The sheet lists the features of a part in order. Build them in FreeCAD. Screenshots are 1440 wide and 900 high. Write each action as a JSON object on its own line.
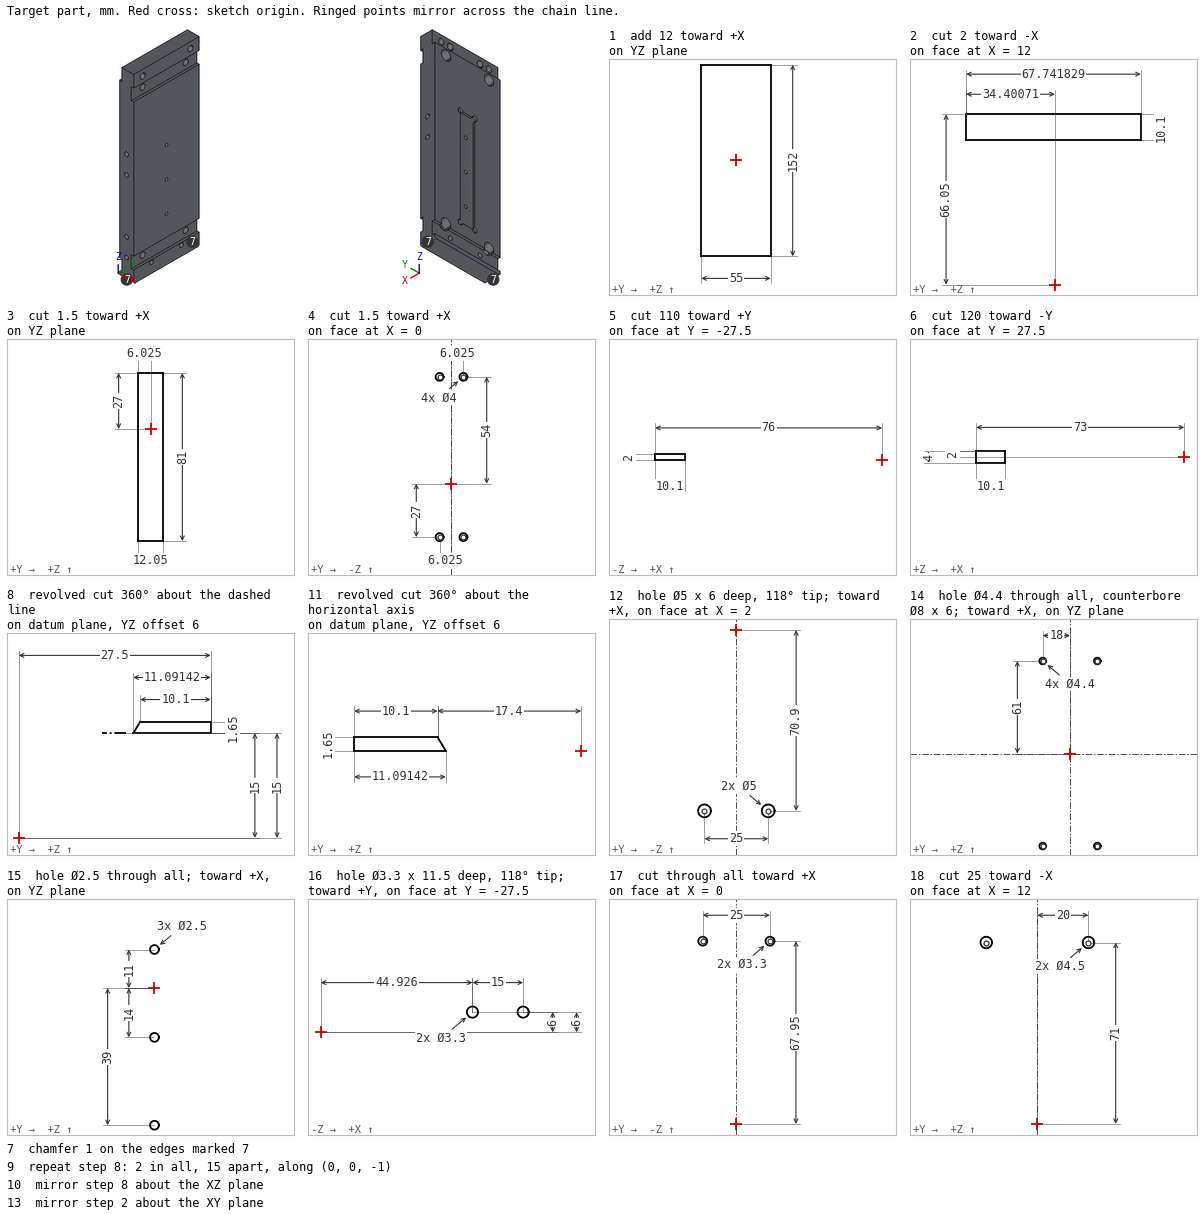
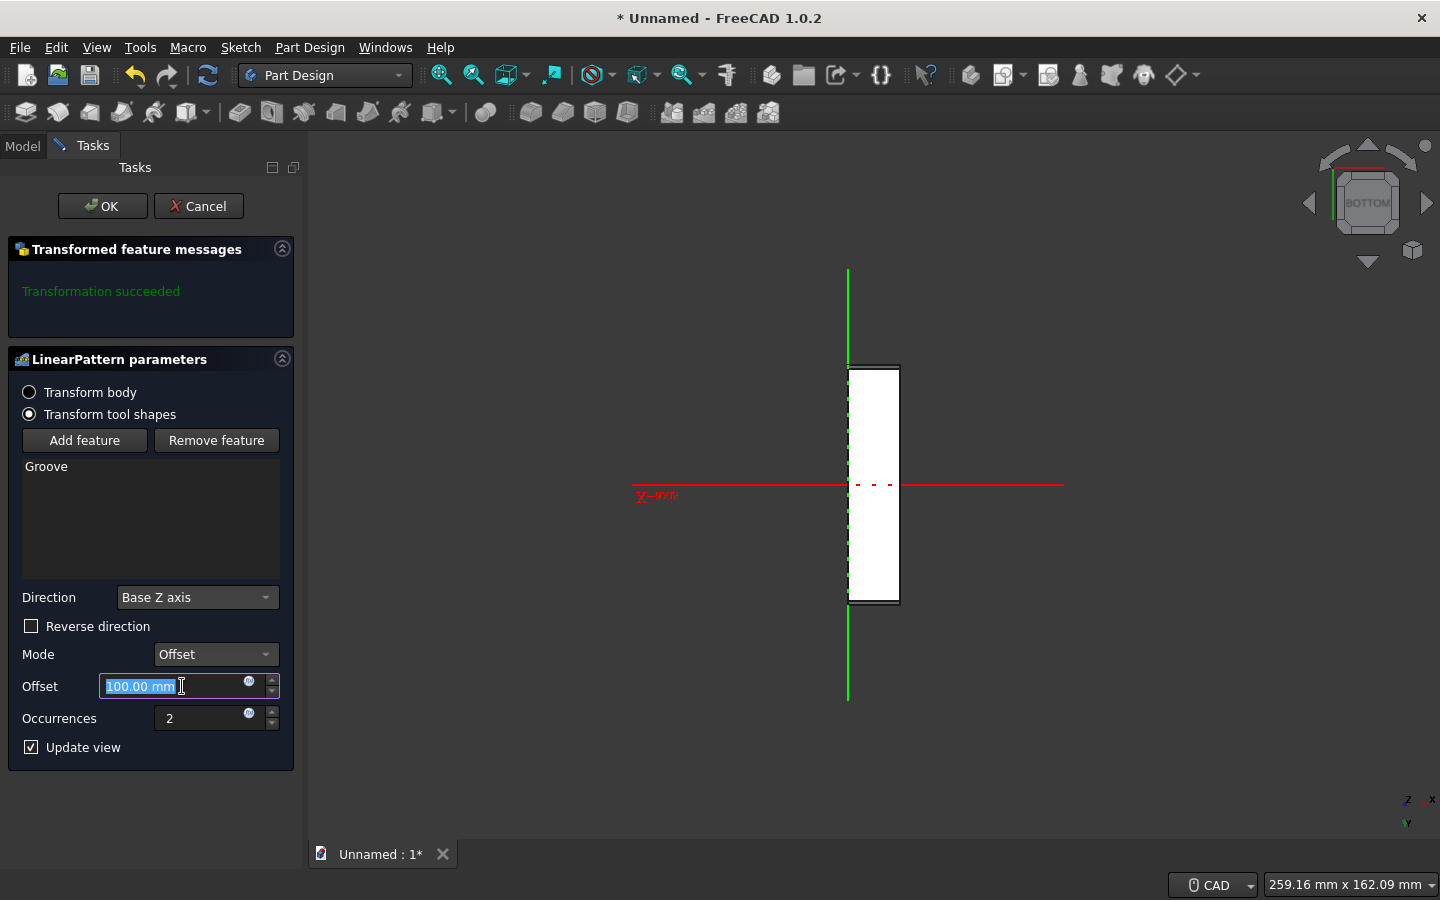
{"action": "type", "text": "15"}
{"action": "key", "text": "Tab"}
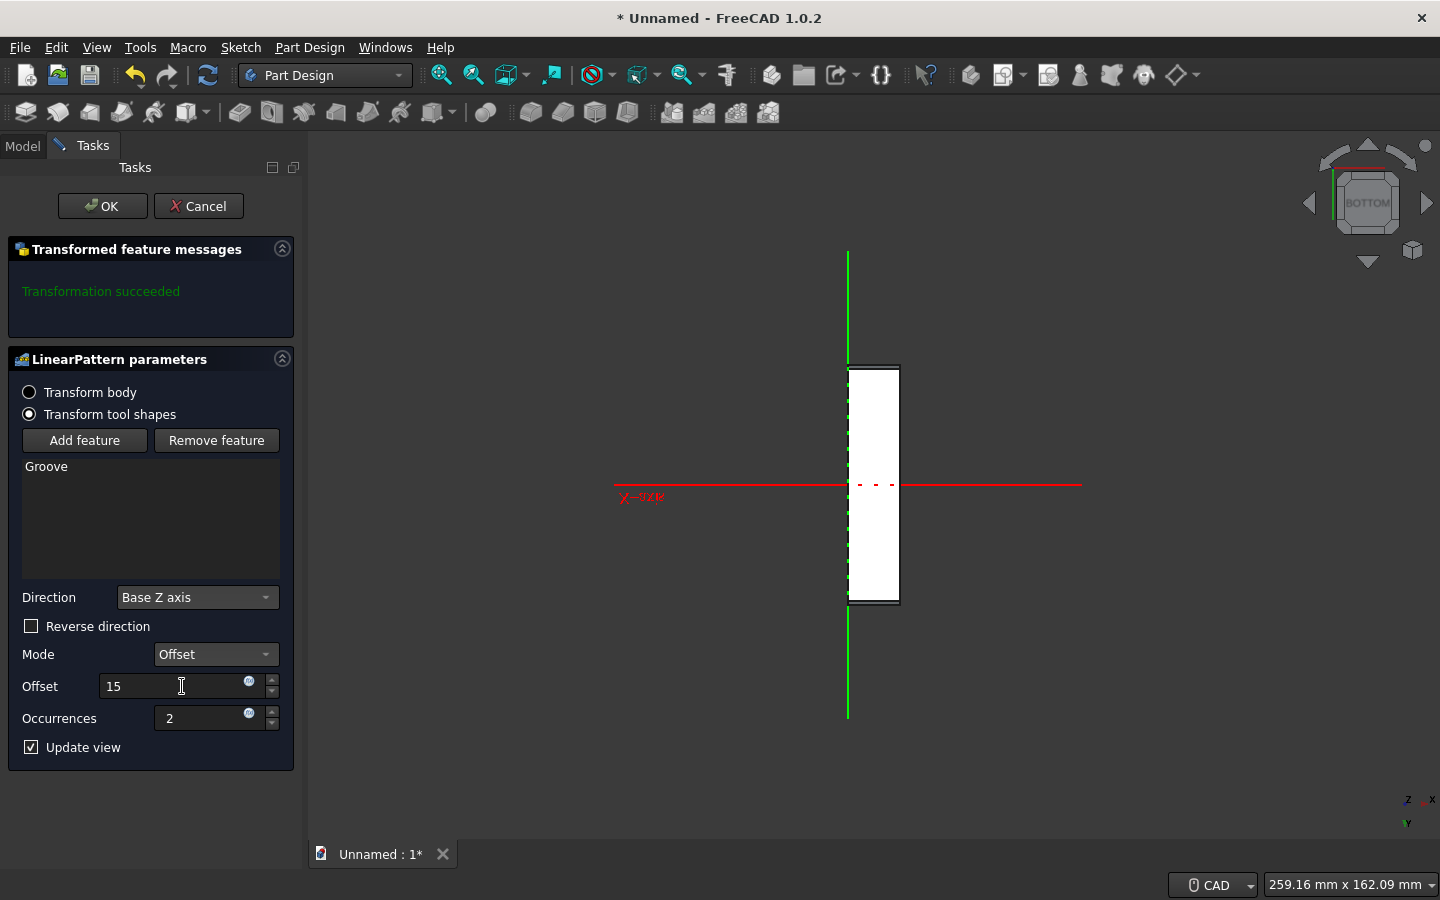
{"action": "triple_click", "coordinate": [209, 718]}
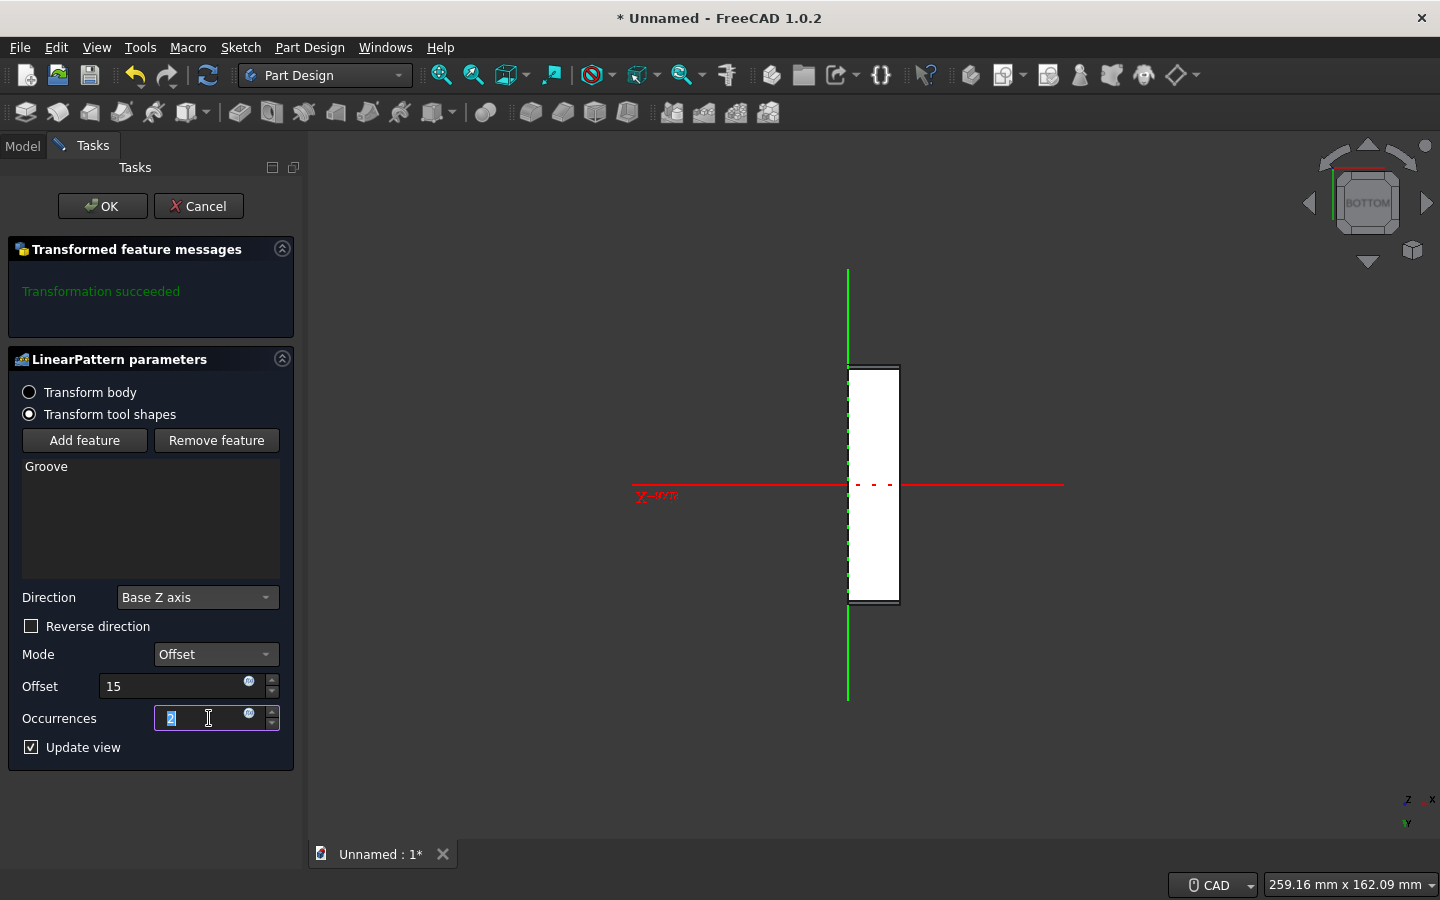
{"action": "type", "text": "2"}
{"action": "key", "text": "Tab"}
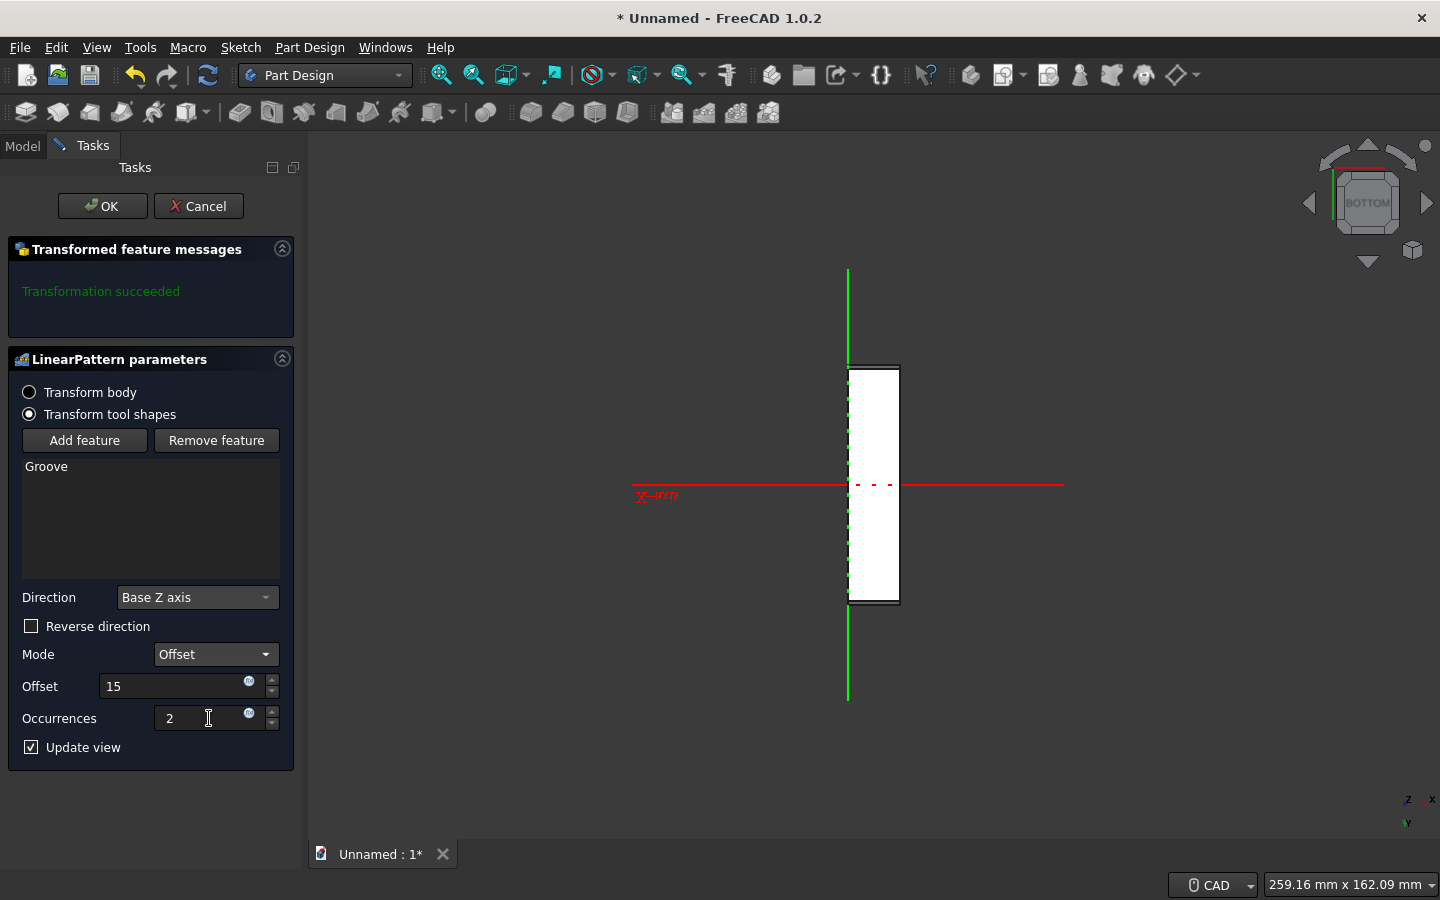
{"action": "left_click", "coordinate": [30, 626]}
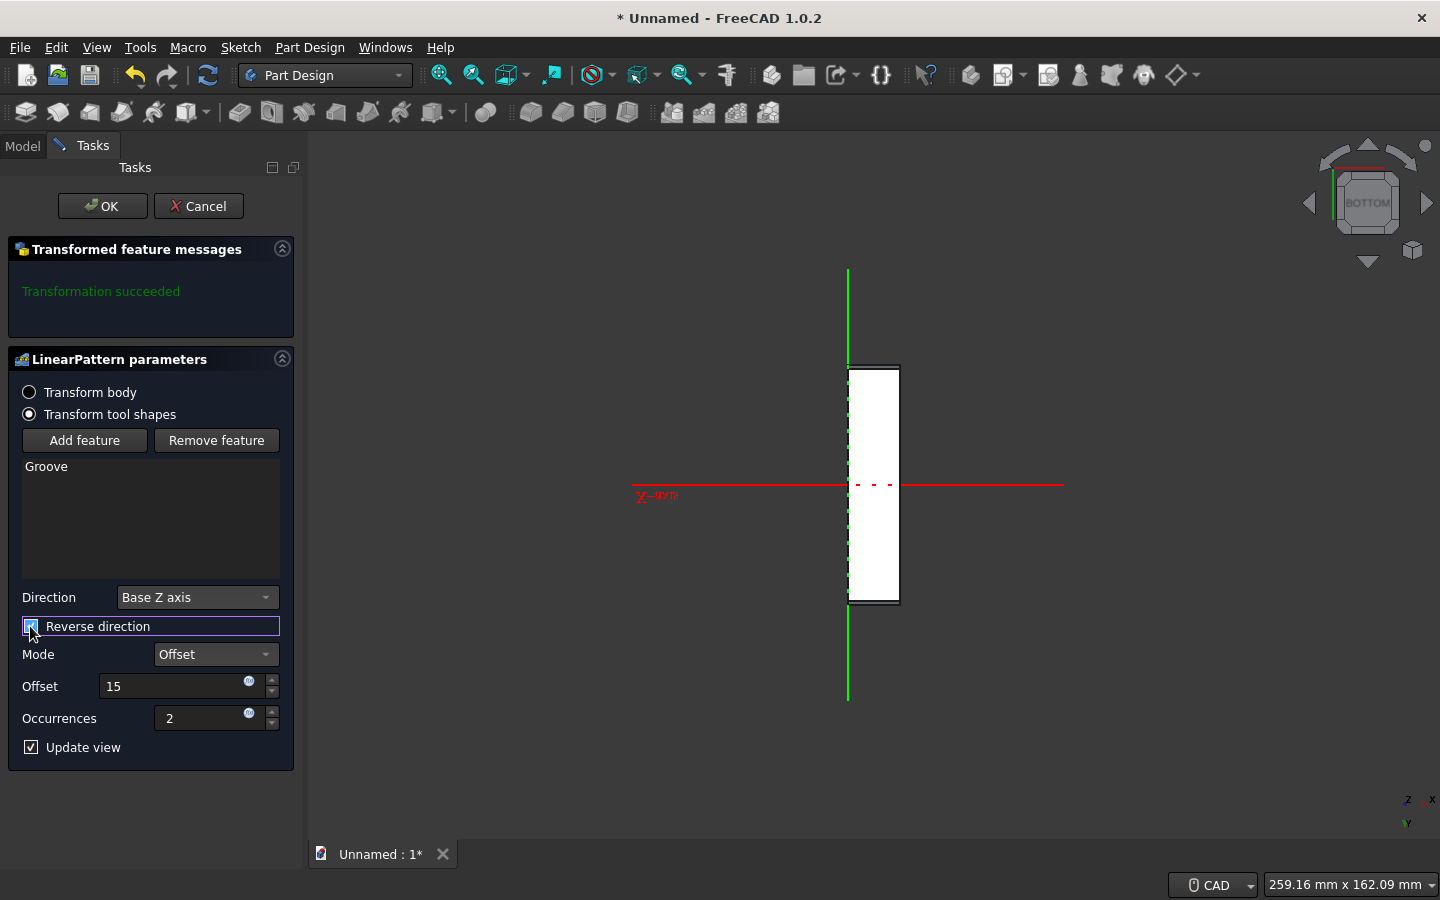
{"action": "left_click", "coordinate": [103, 206]}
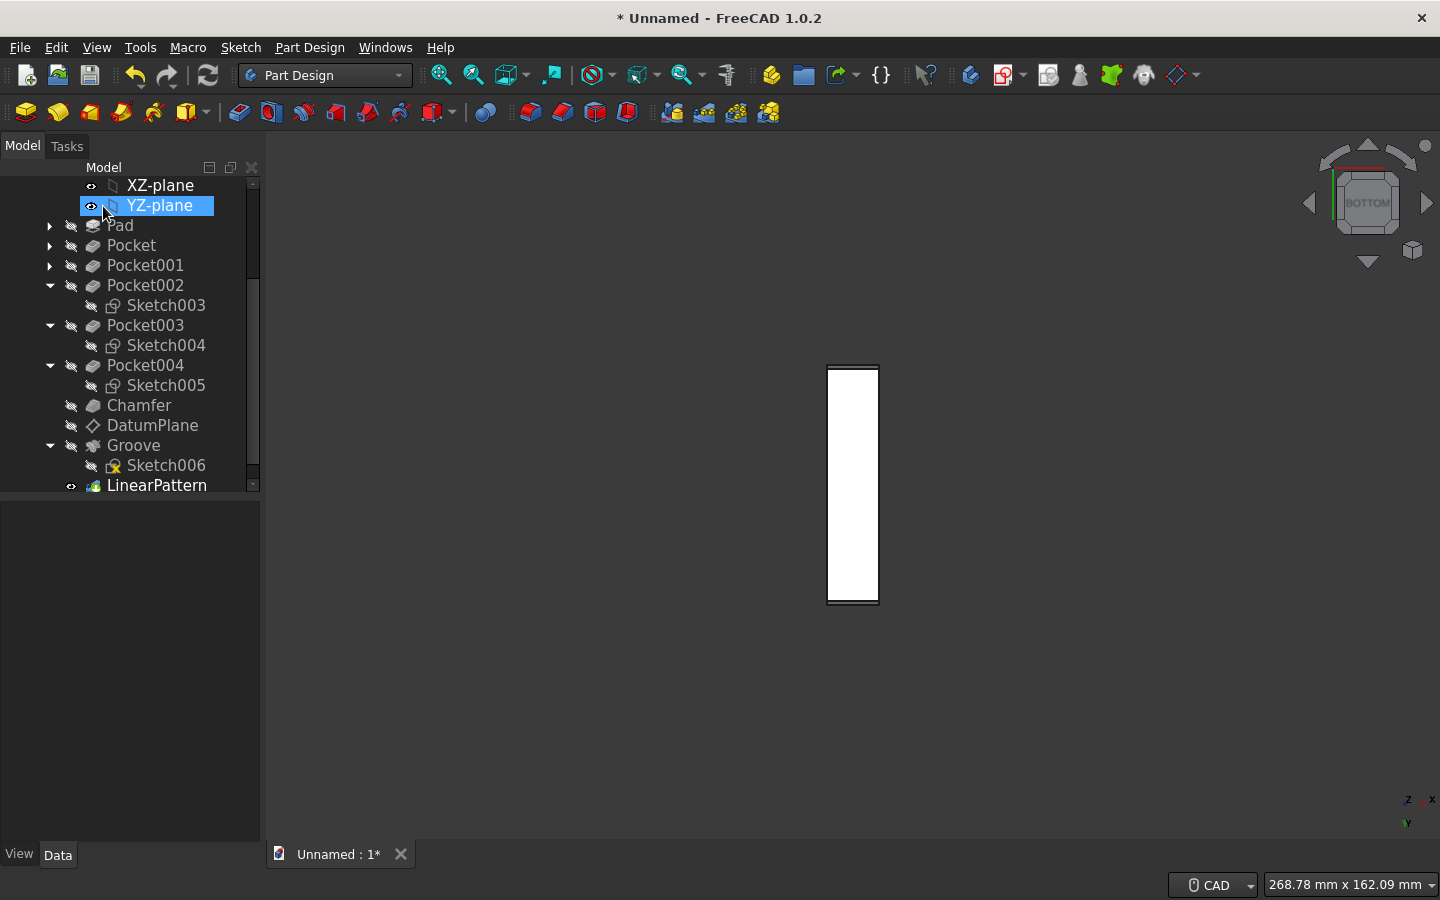
{"action": "left_click", "coordinate": [442, 76]}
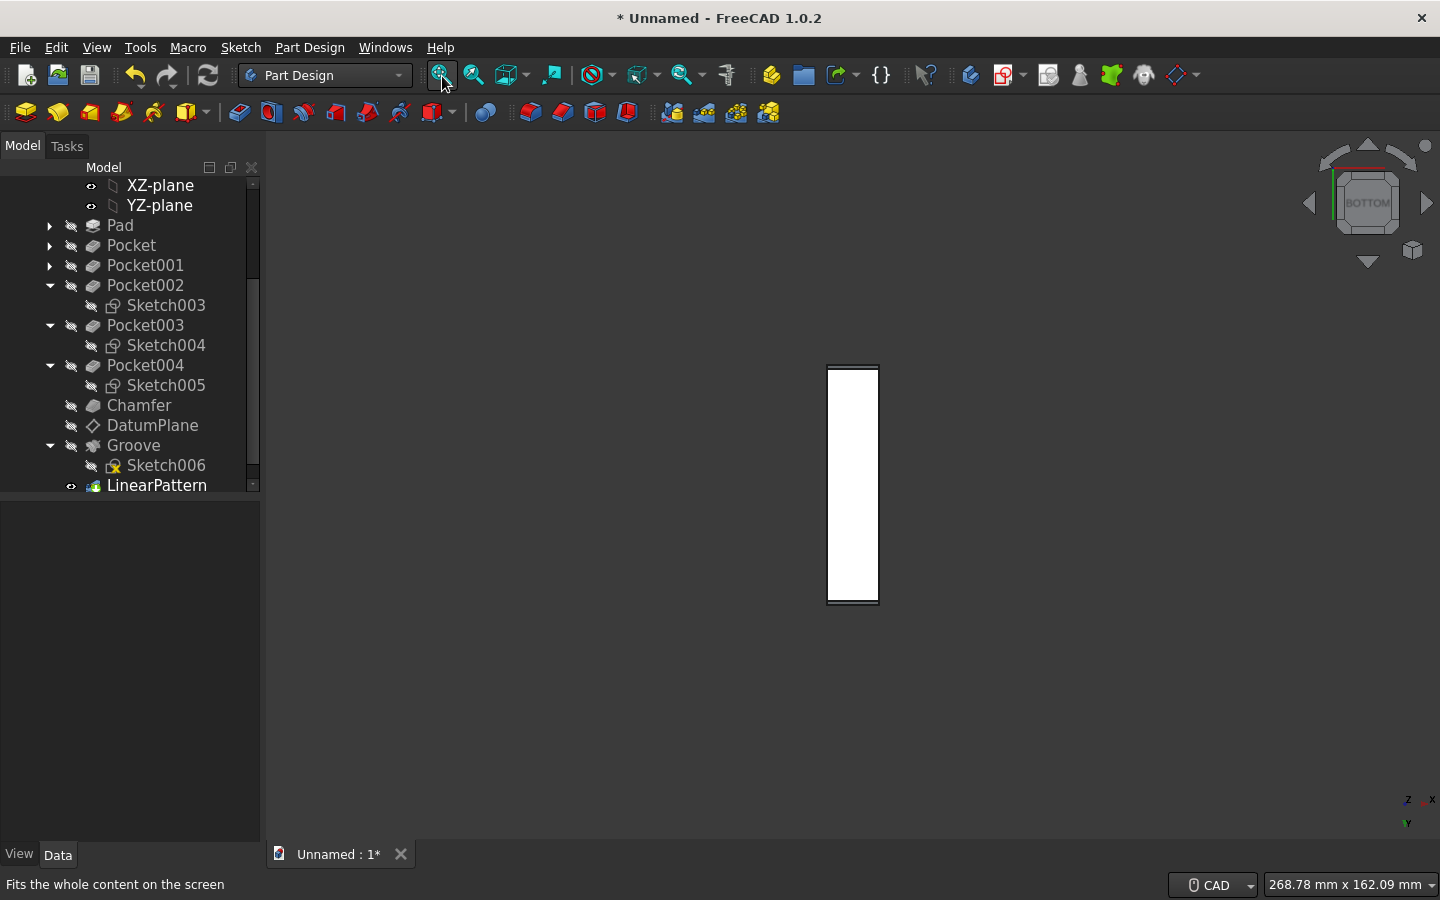
{"action": "left_click", "coordinate": [116, 446]}